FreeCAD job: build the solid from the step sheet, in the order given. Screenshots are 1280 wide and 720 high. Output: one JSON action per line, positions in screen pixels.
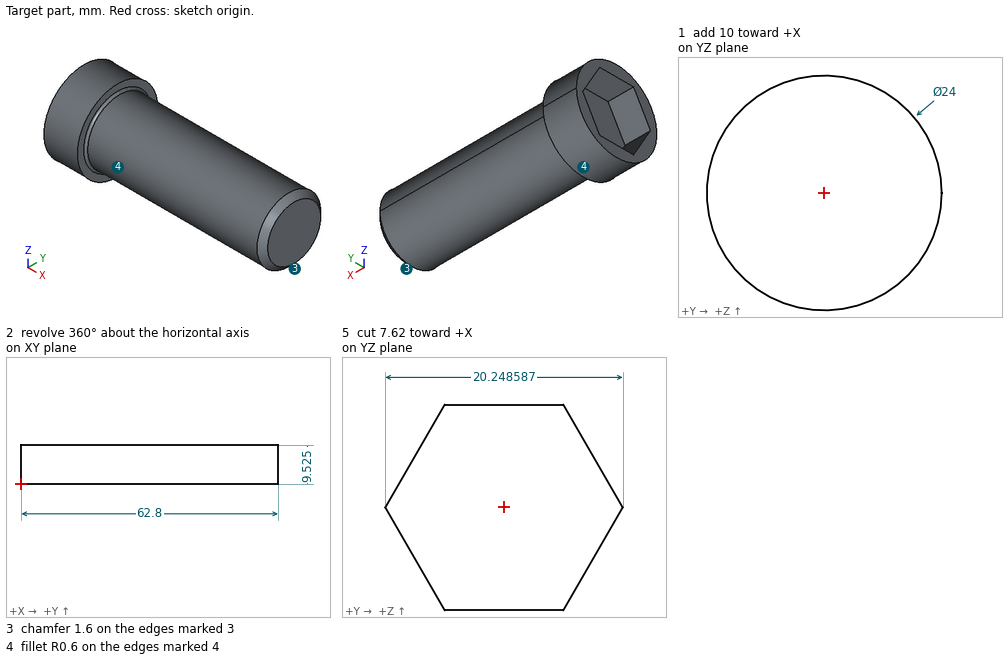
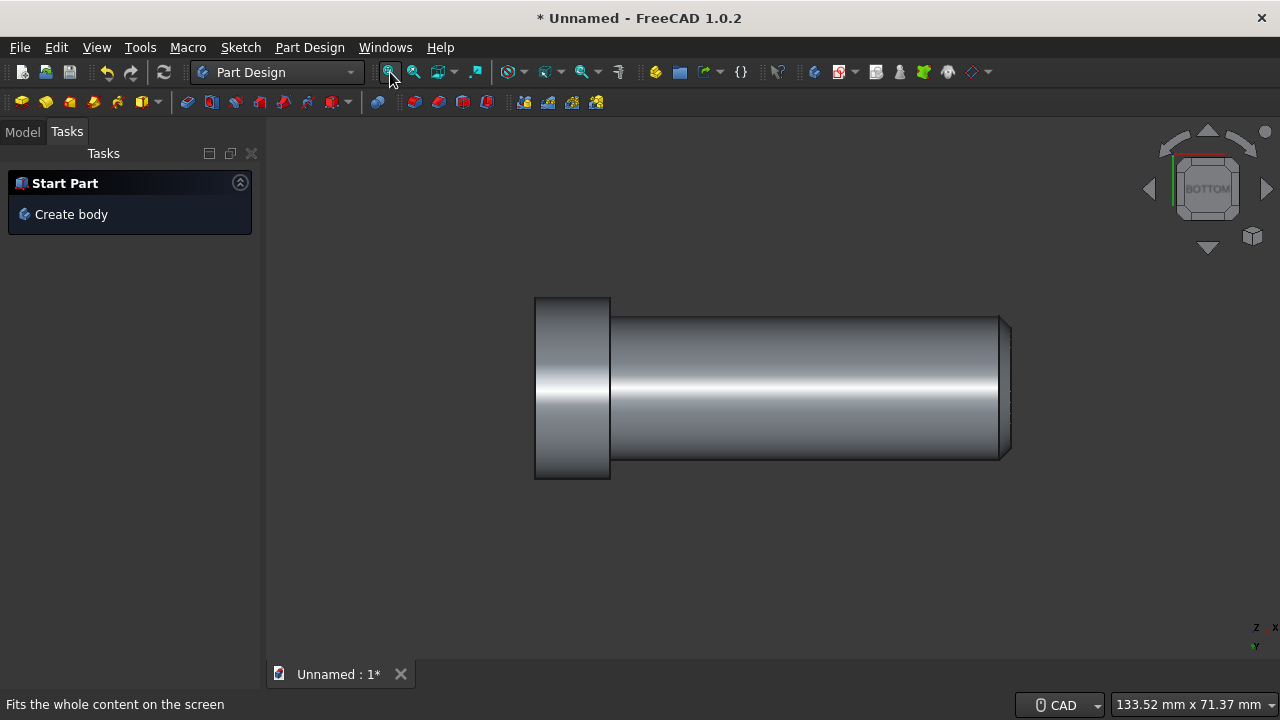
{"action": "key", "text": "4"}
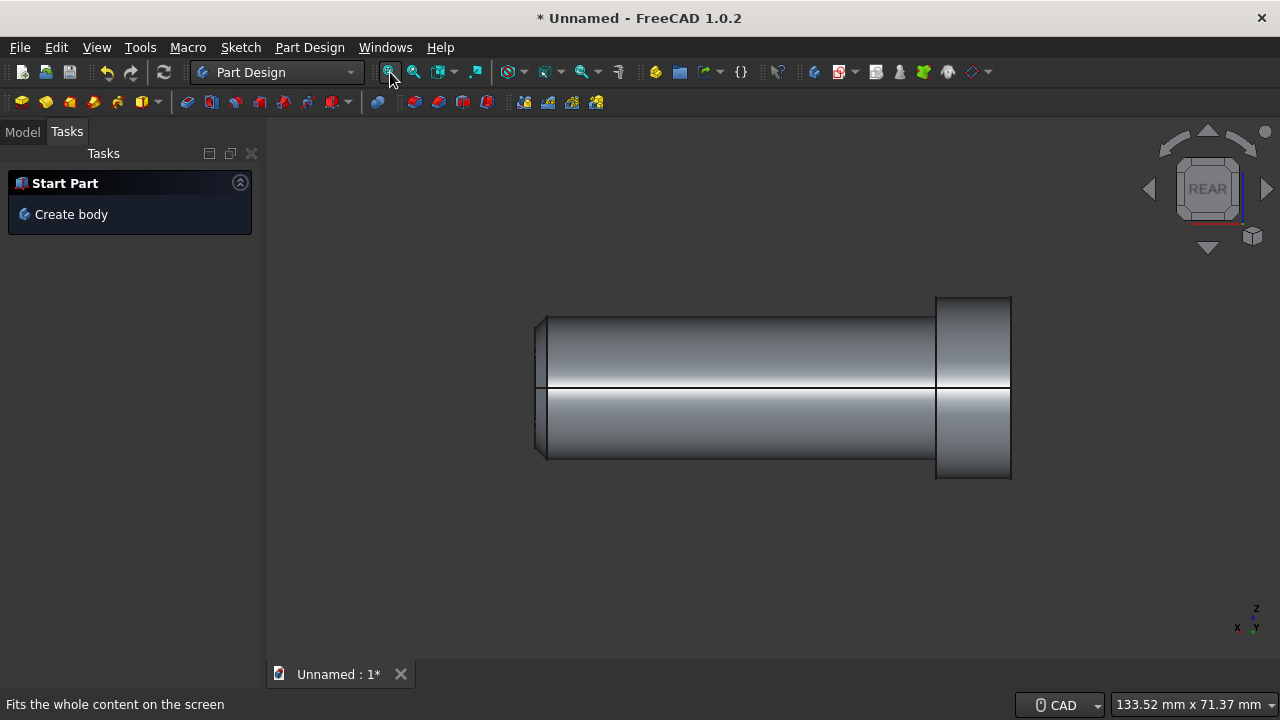
{"action": "key", "text": "6"}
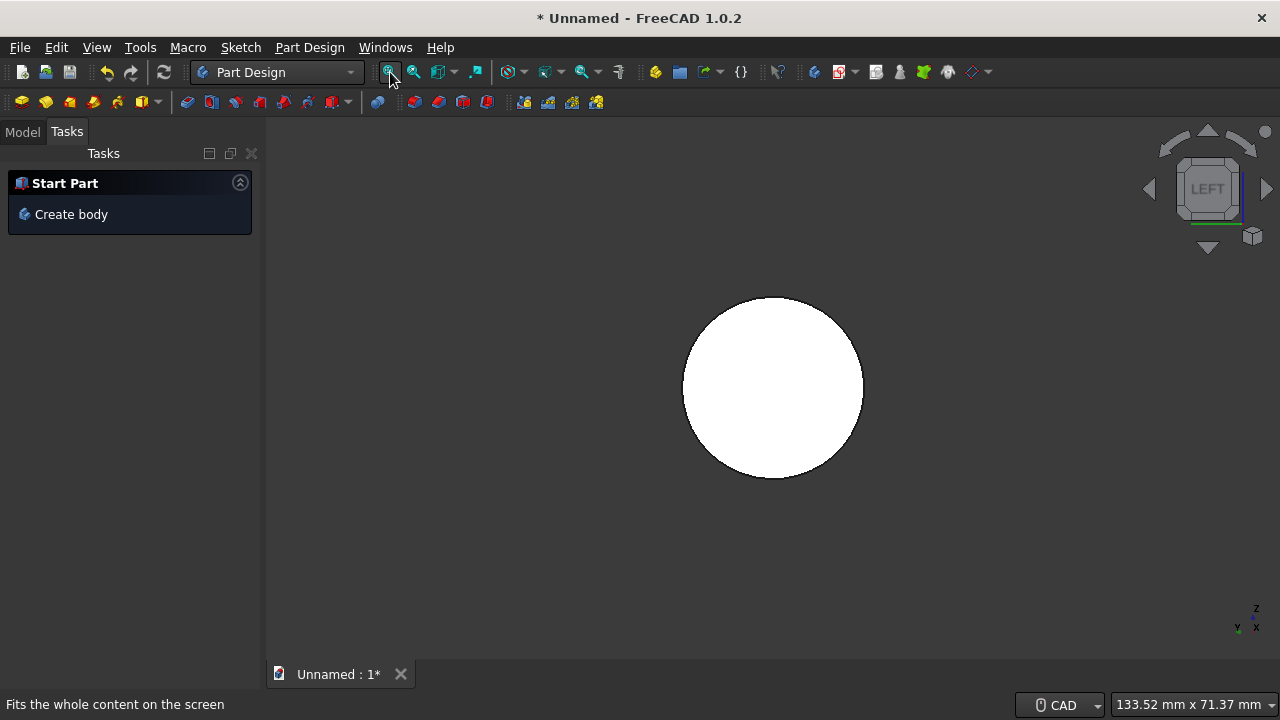
{"action": "left_click", "coordinate": [390, 72]}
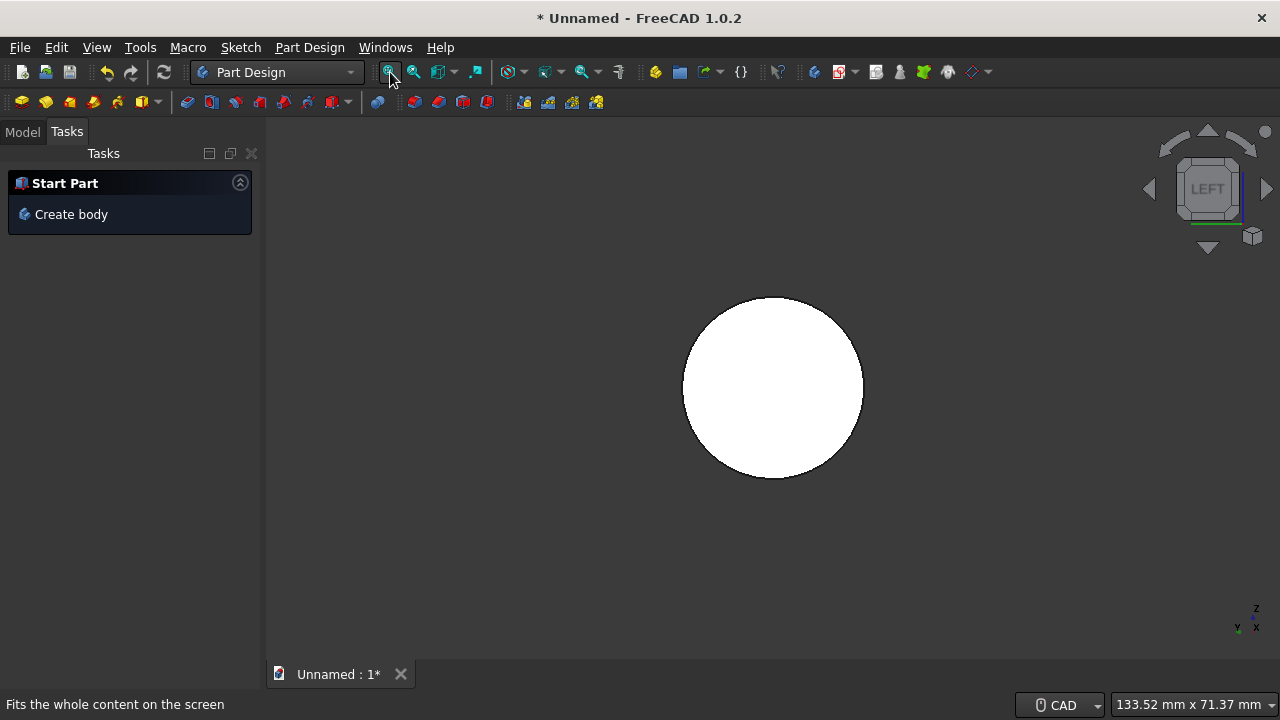
{"action": "key", "text": "v 3"}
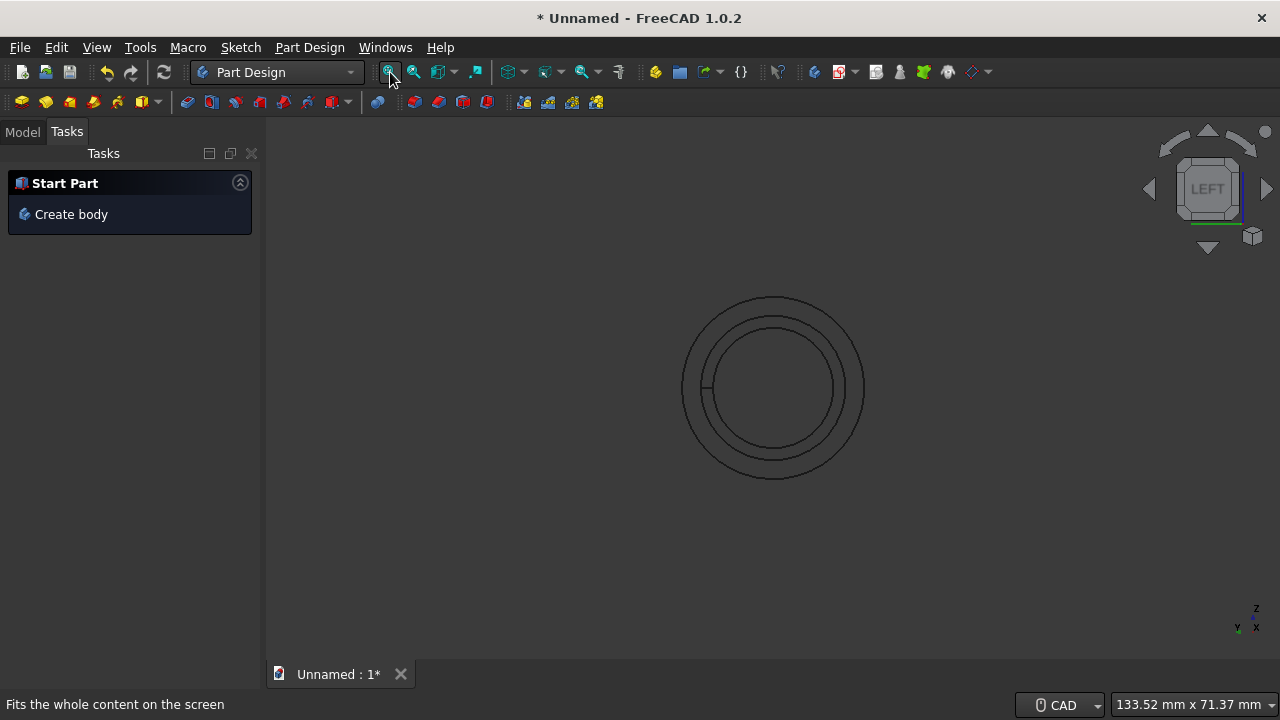
{"action": "key", "text": "0"}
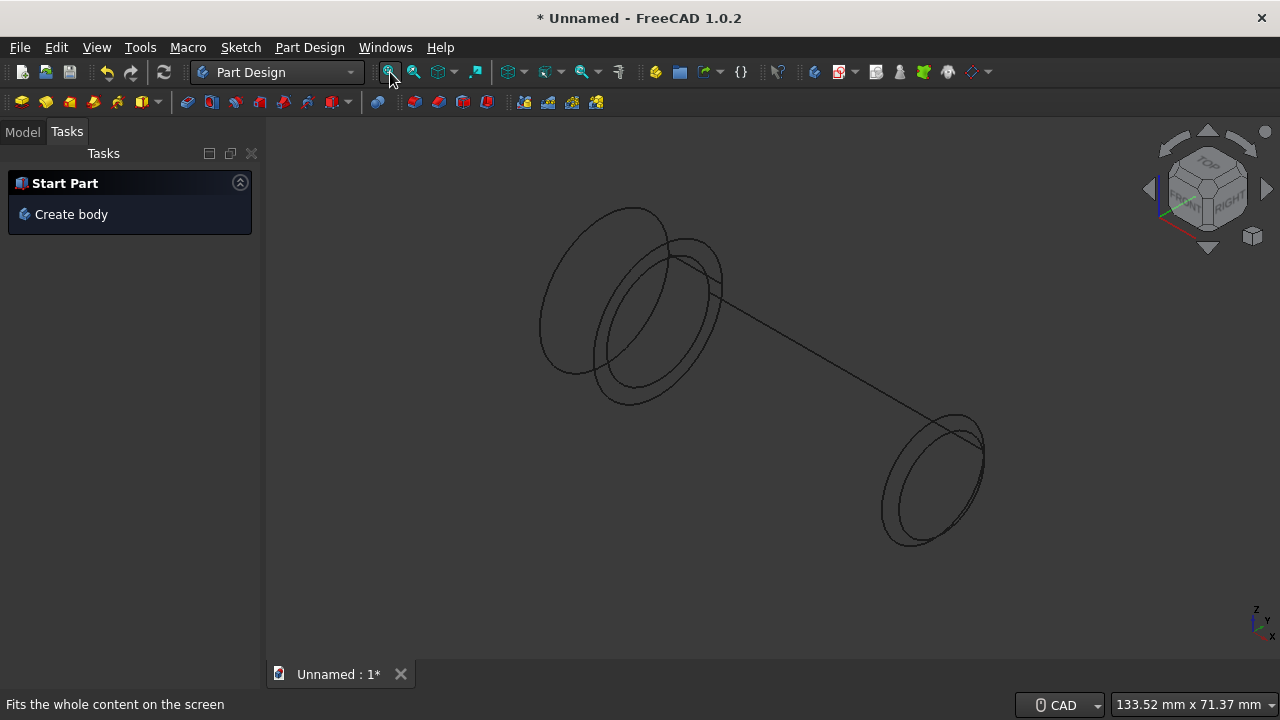
{"action": "left_click", "coordinate": [607, 350]}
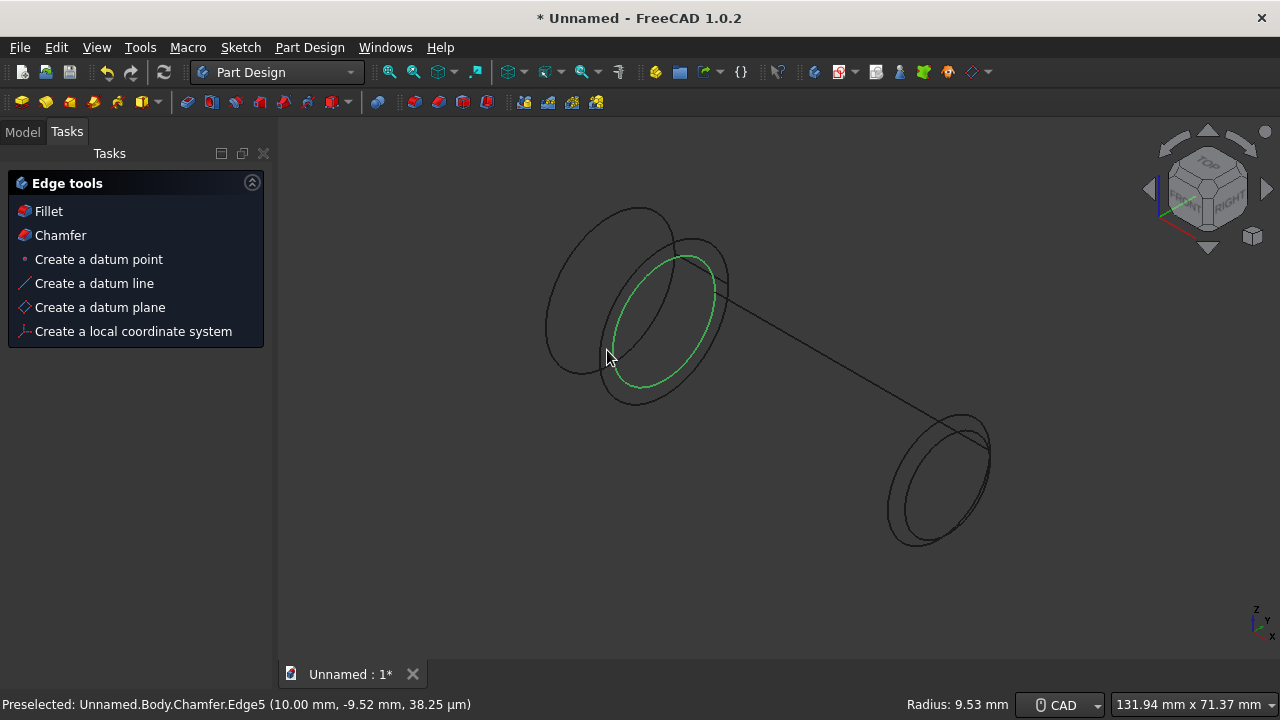
{"action": "key", "text": "v 1"}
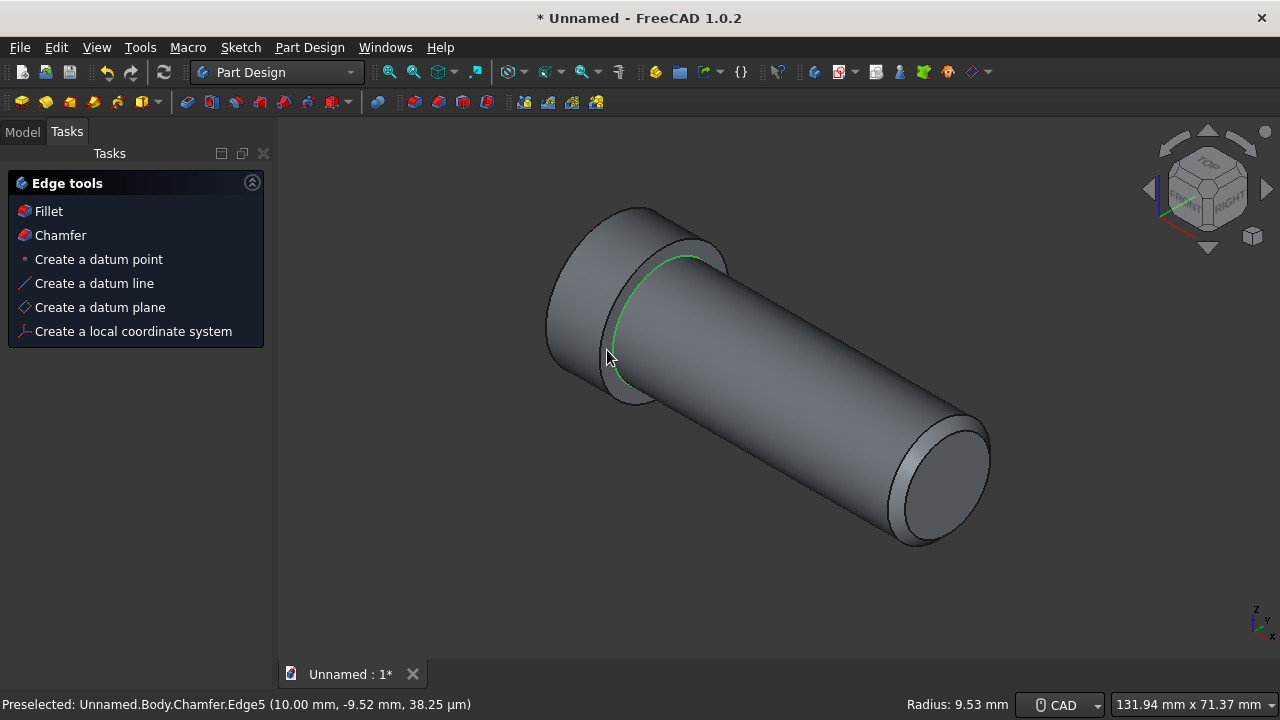
{"action": "left_click", "coordinate": [416, 102]}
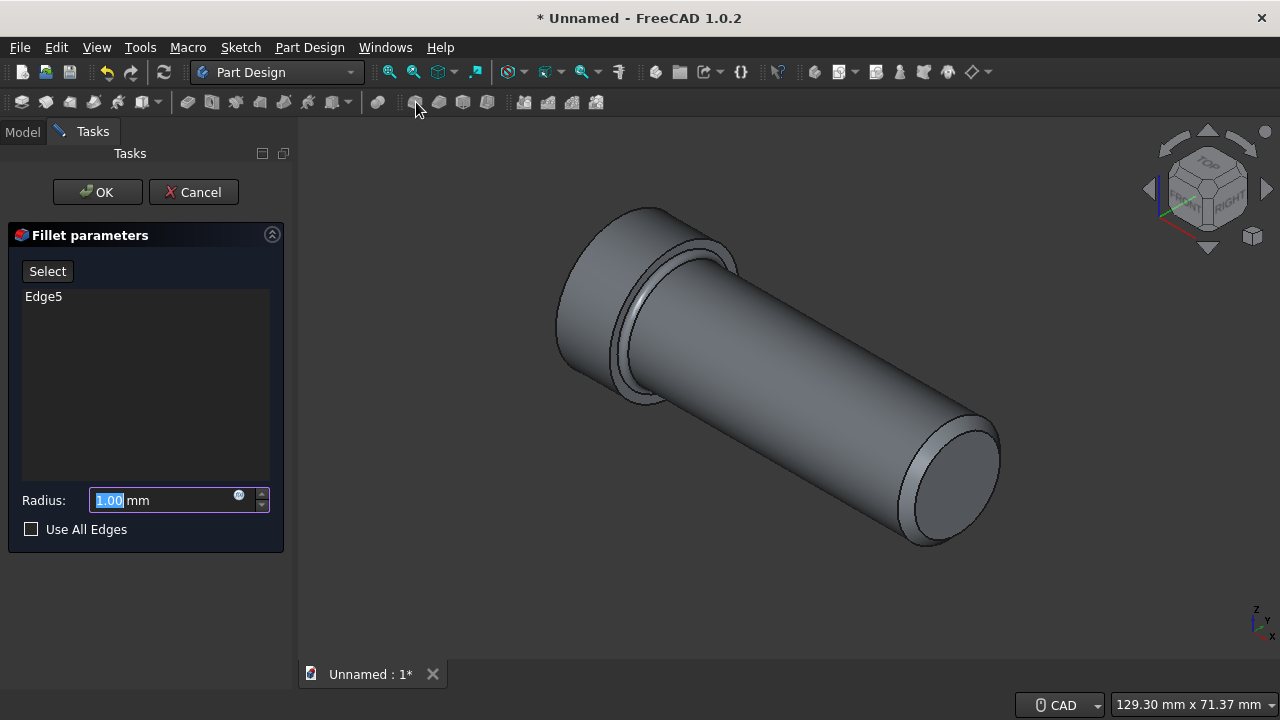
{"action": "type", "text": "0.6"}
{"action": "key", "text": "Tab"}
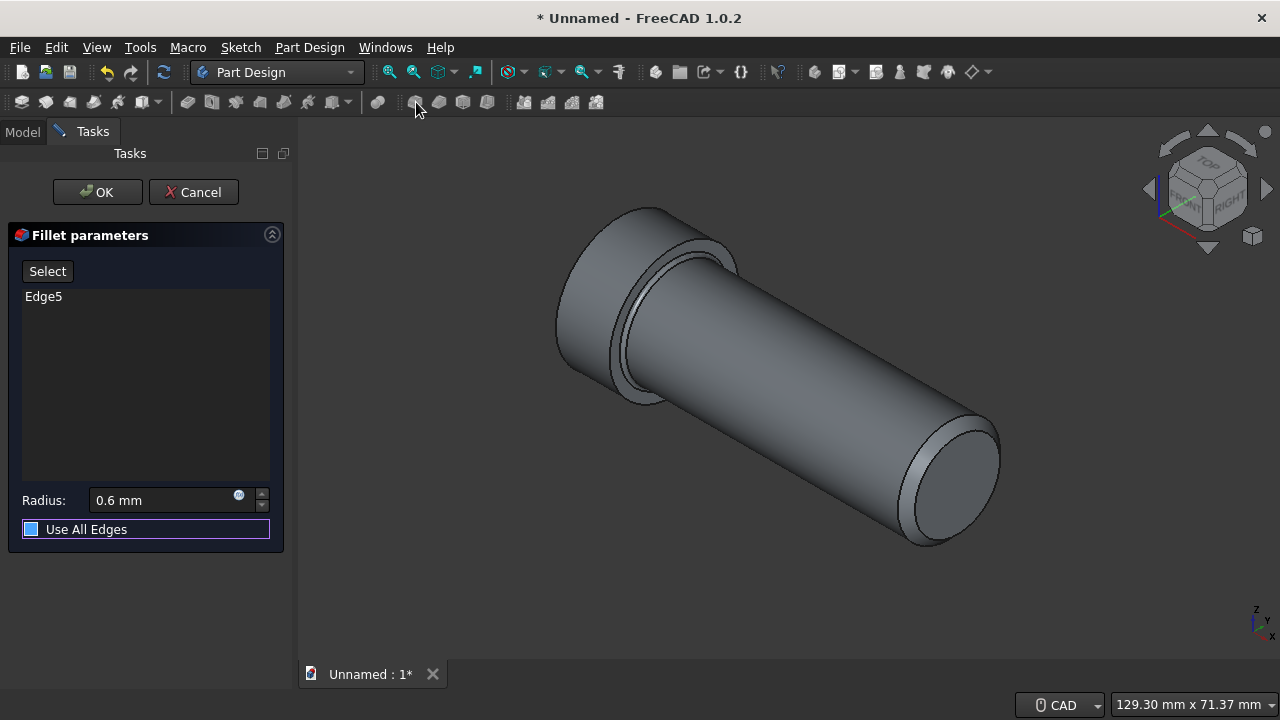
{"action": "left_click", "coordinate": [98, 192]}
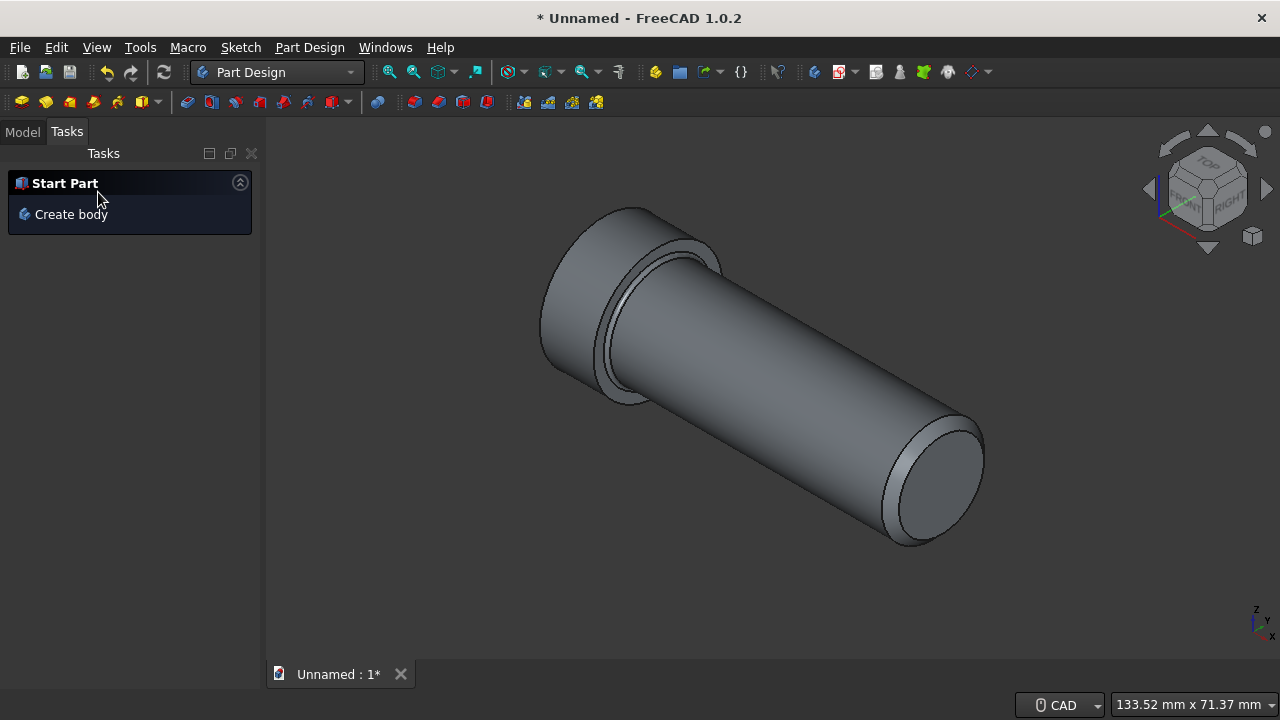
{"action": "left_click", "coordinate": [840, 72]}